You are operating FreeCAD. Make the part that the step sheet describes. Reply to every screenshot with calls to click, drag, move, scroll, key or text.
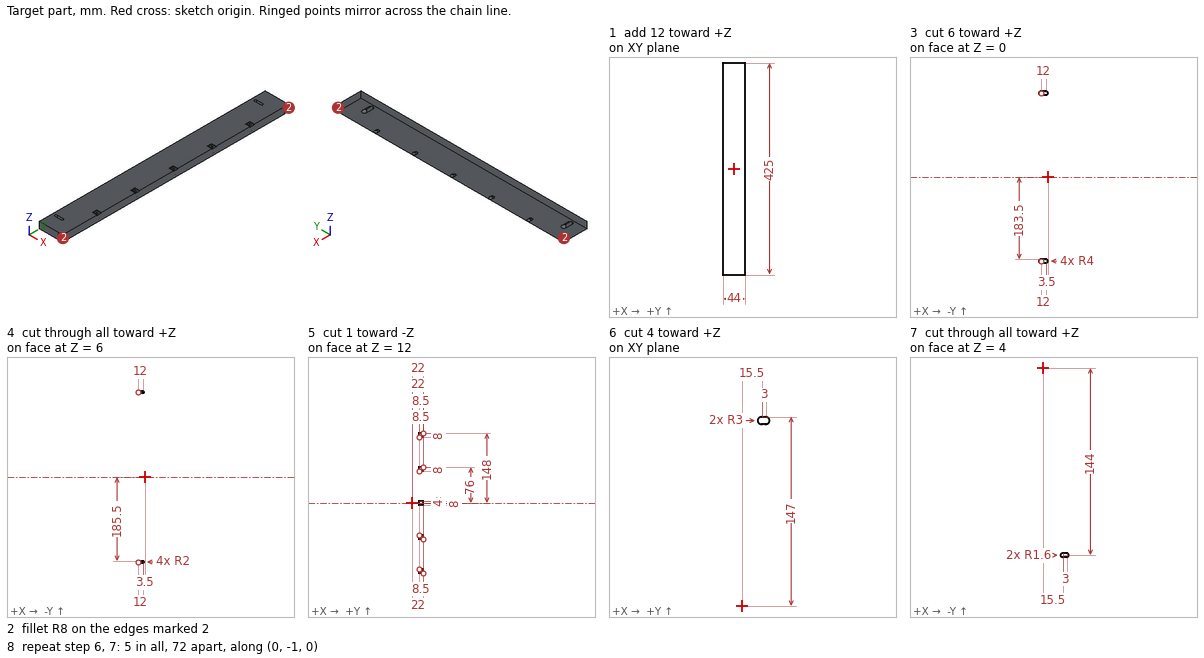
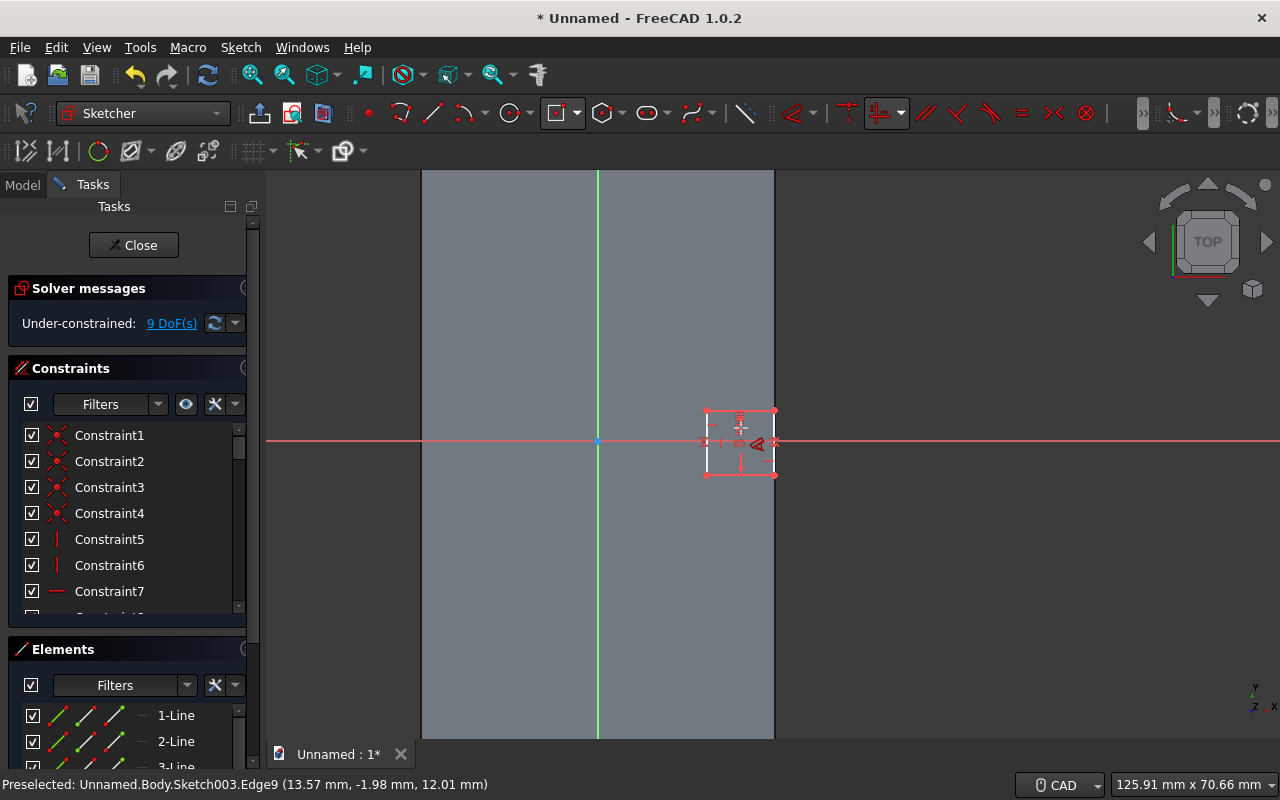
scroll(707, 411, up, 2)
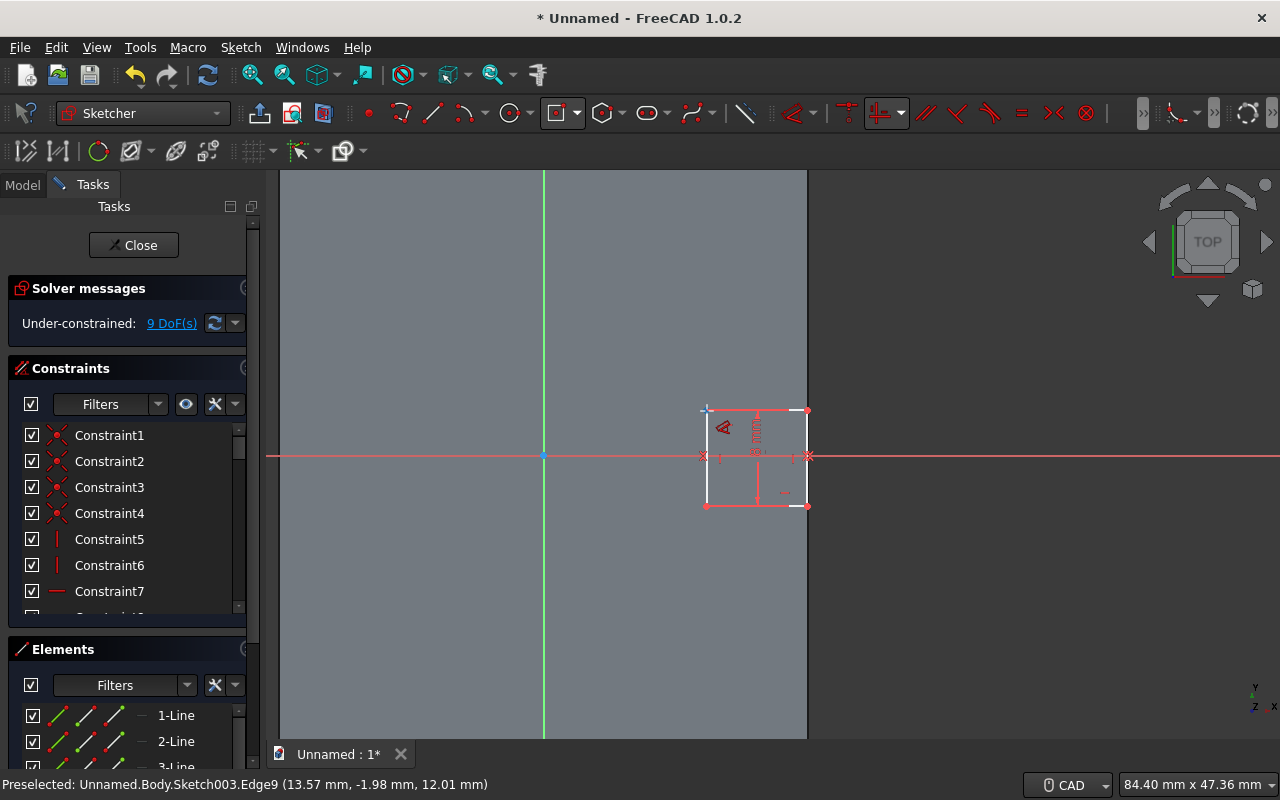
click(707, 410)
click(510, 433)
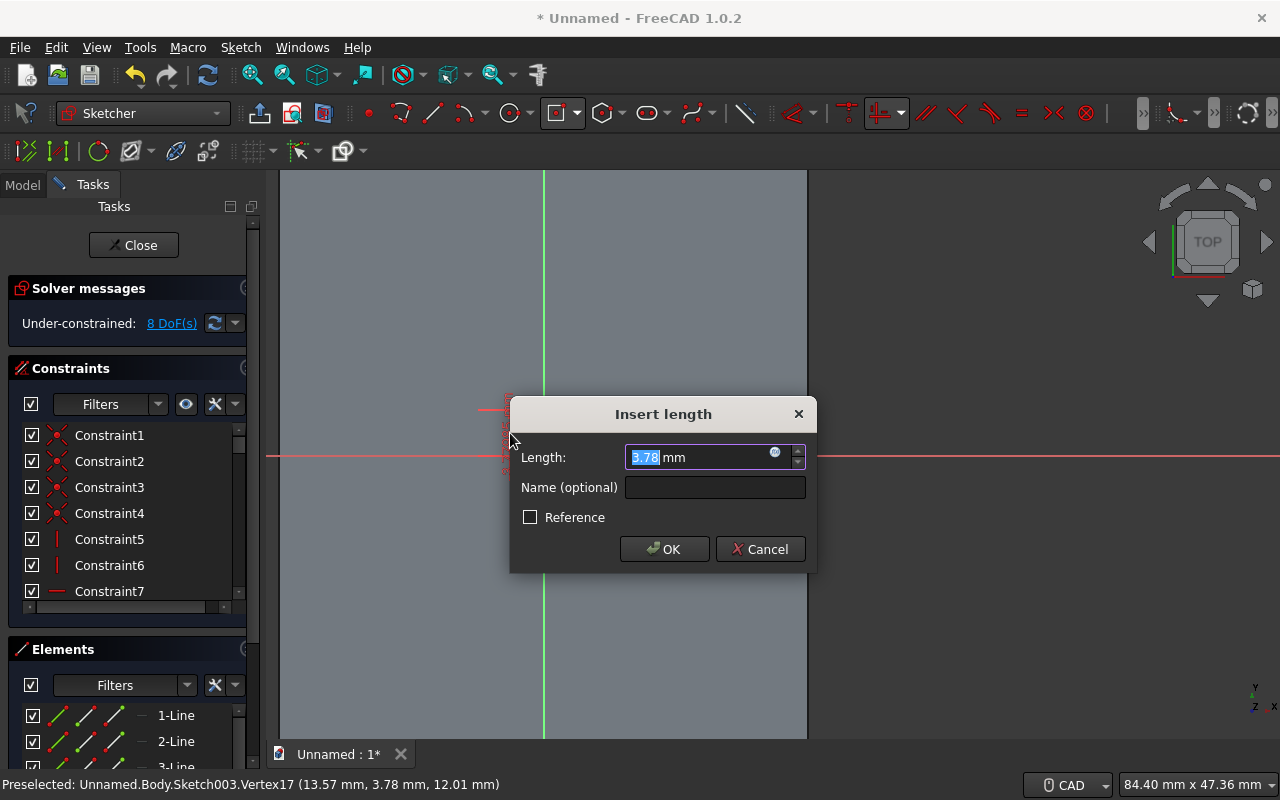
text(4)
key(Return)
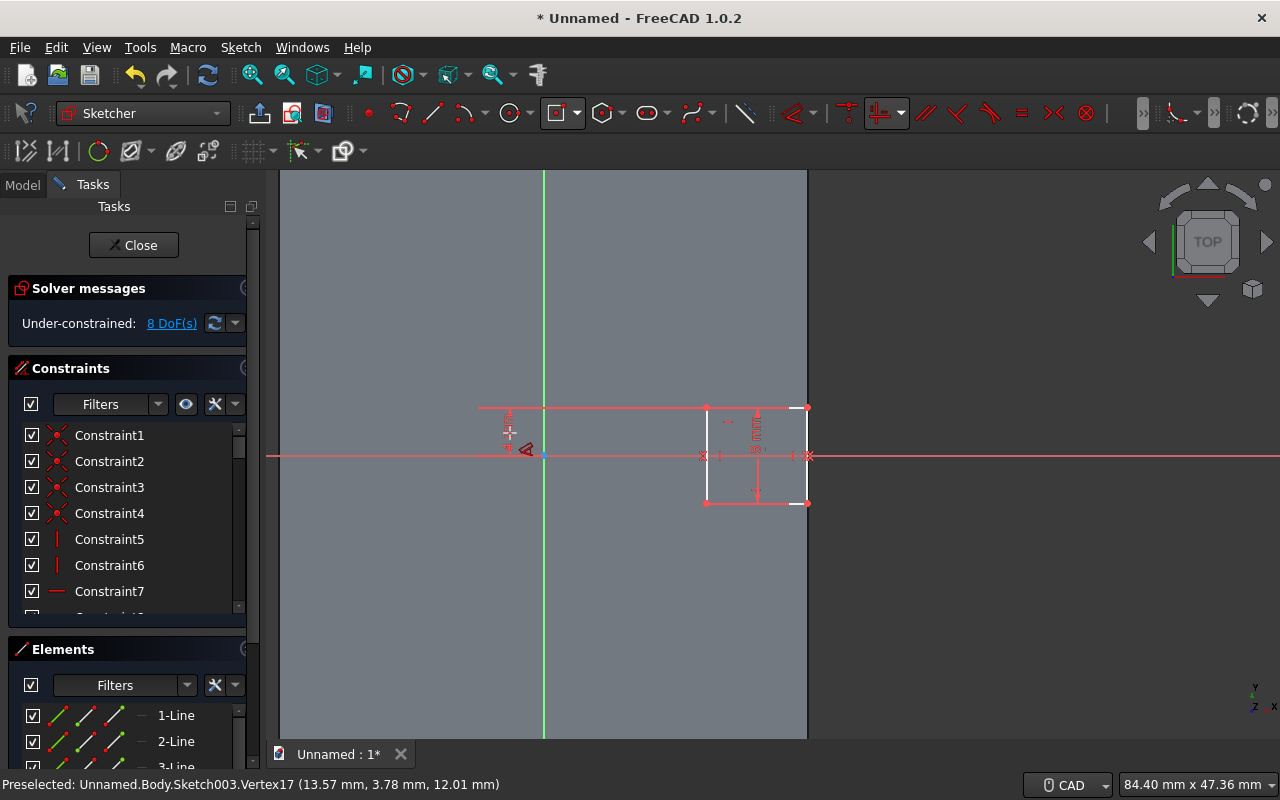
scroll(708, 454, down, 11)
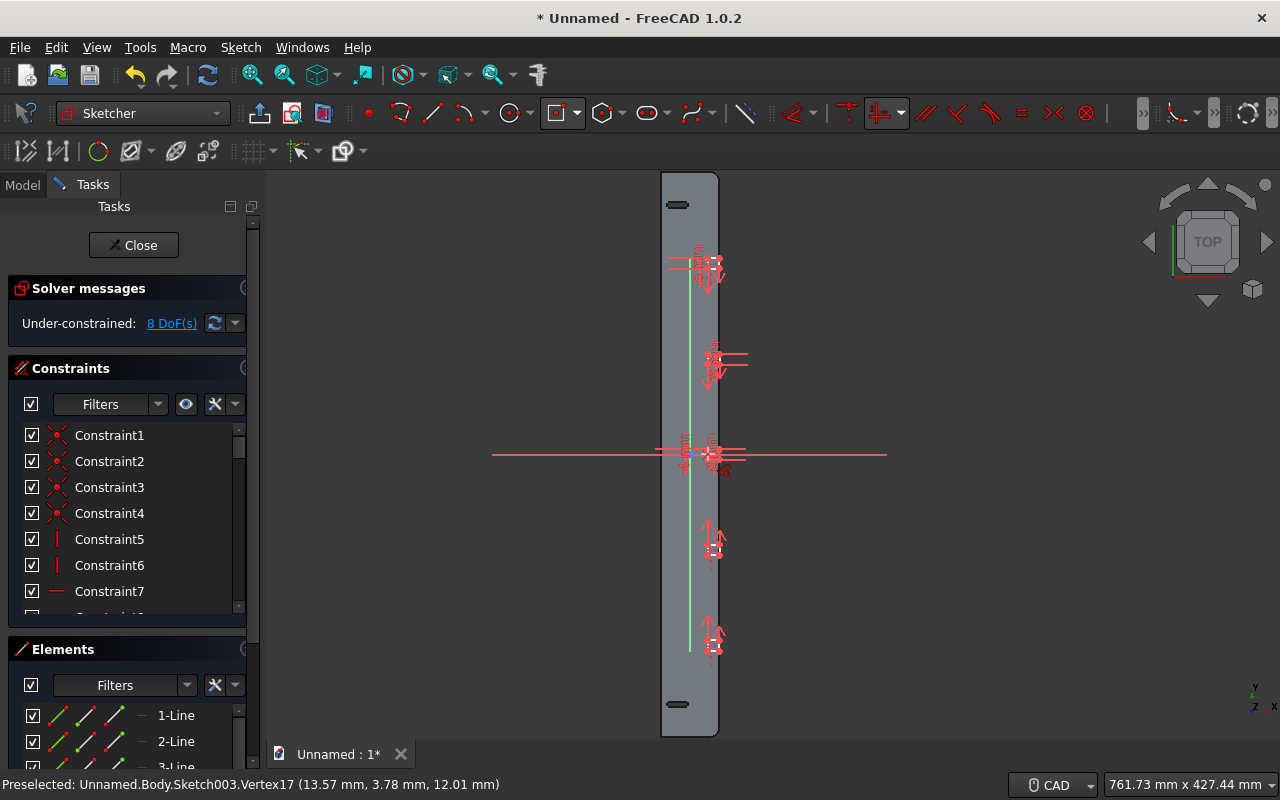
scroll(711, 269, up, 7)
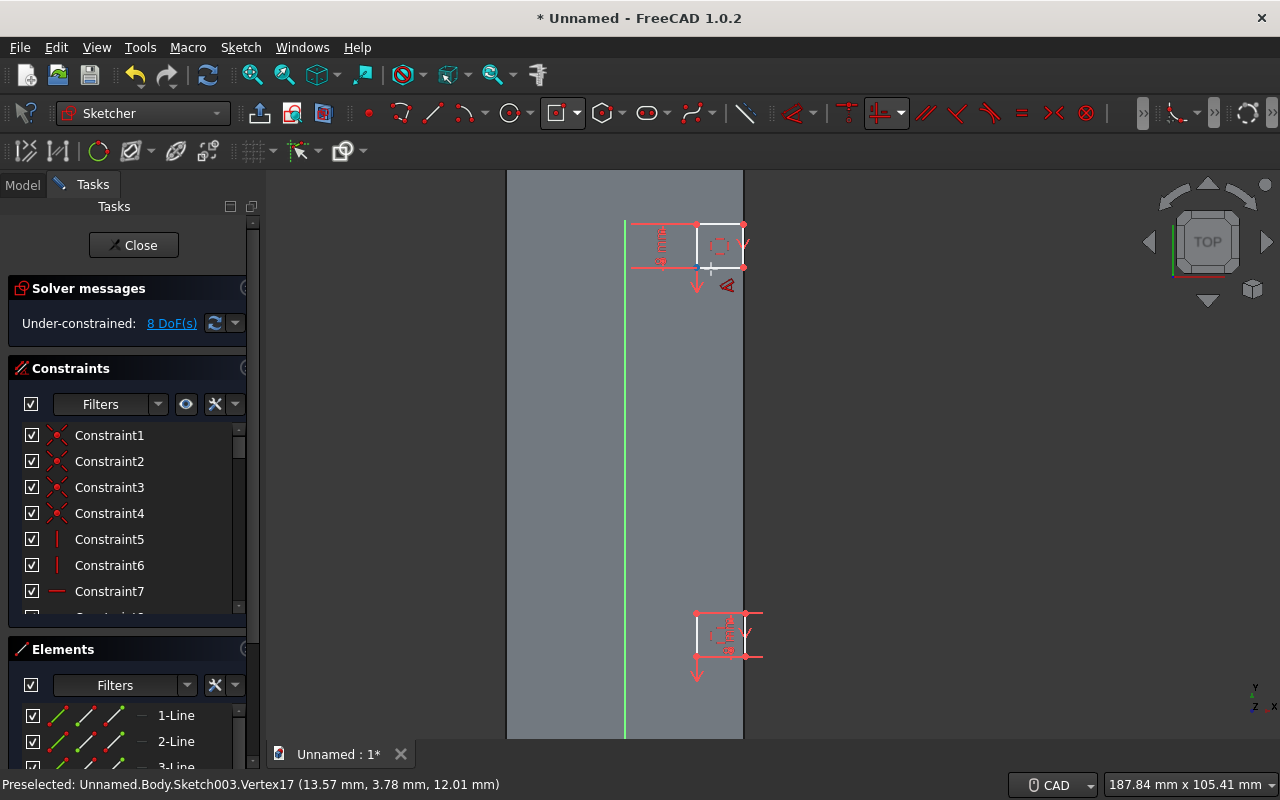
click(711, 268)
click(720, 302)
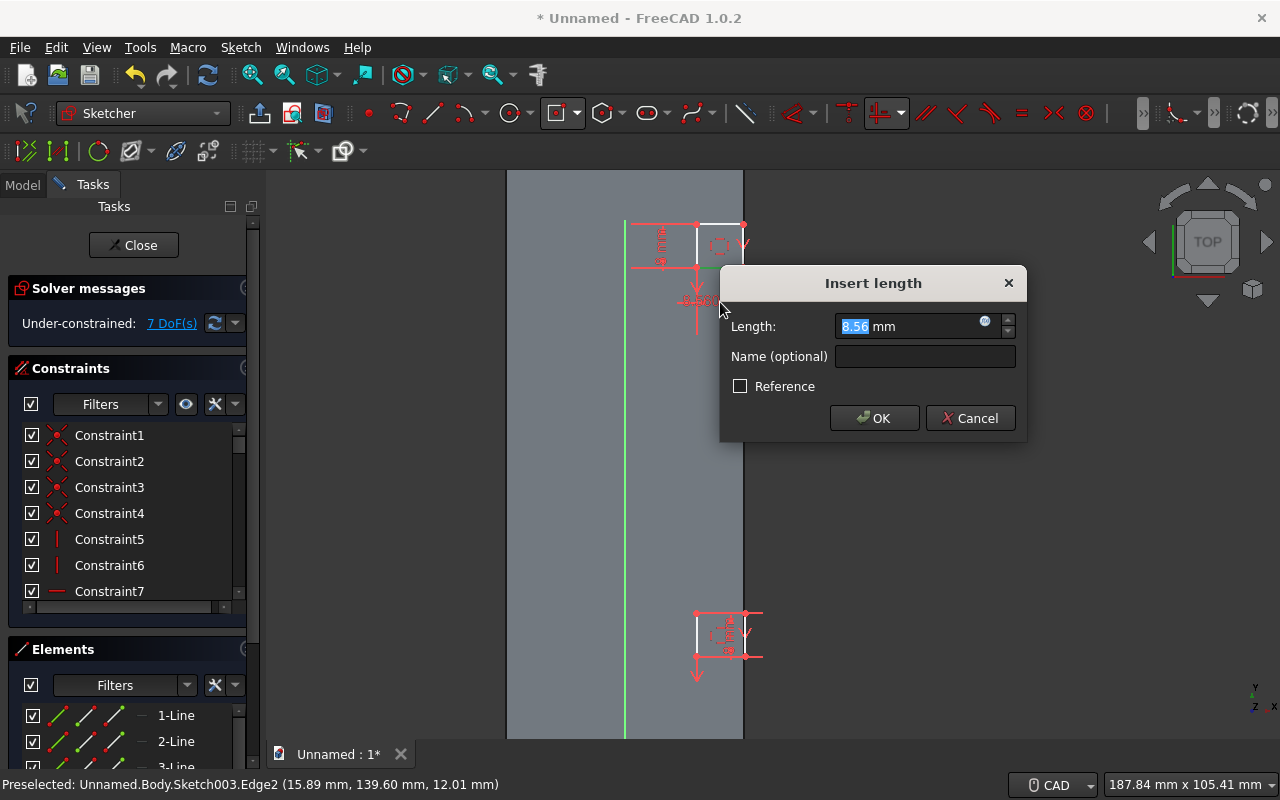
text(8.5)
key(Return)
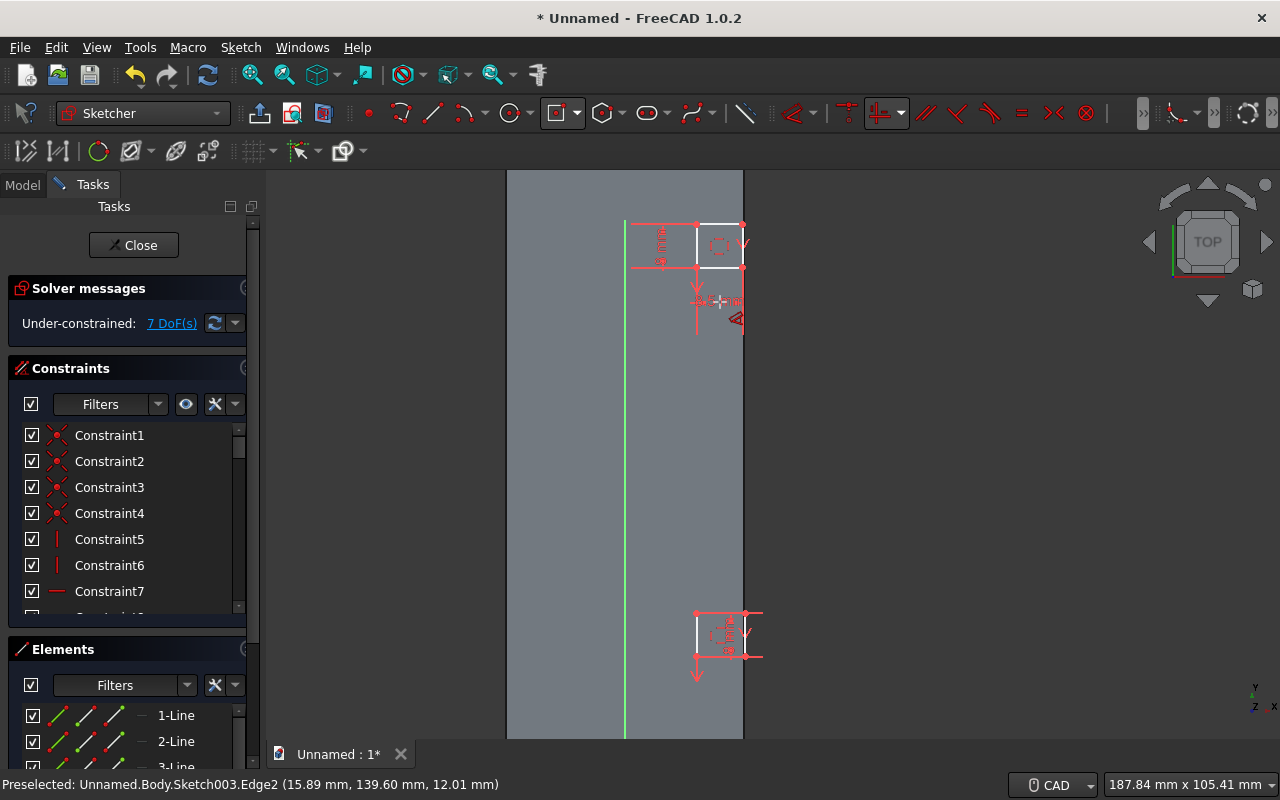
click(711, 657)
click(721, 691)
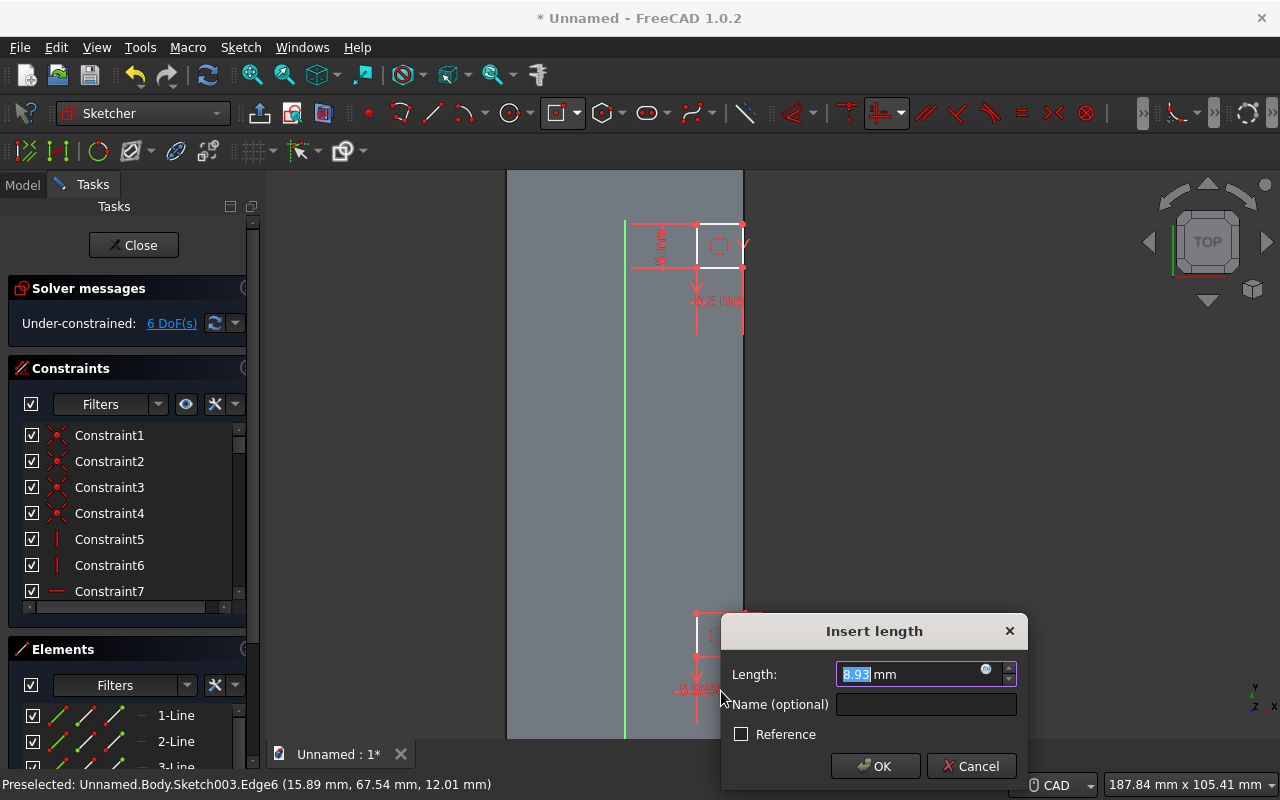
text(8.5)
key(Return)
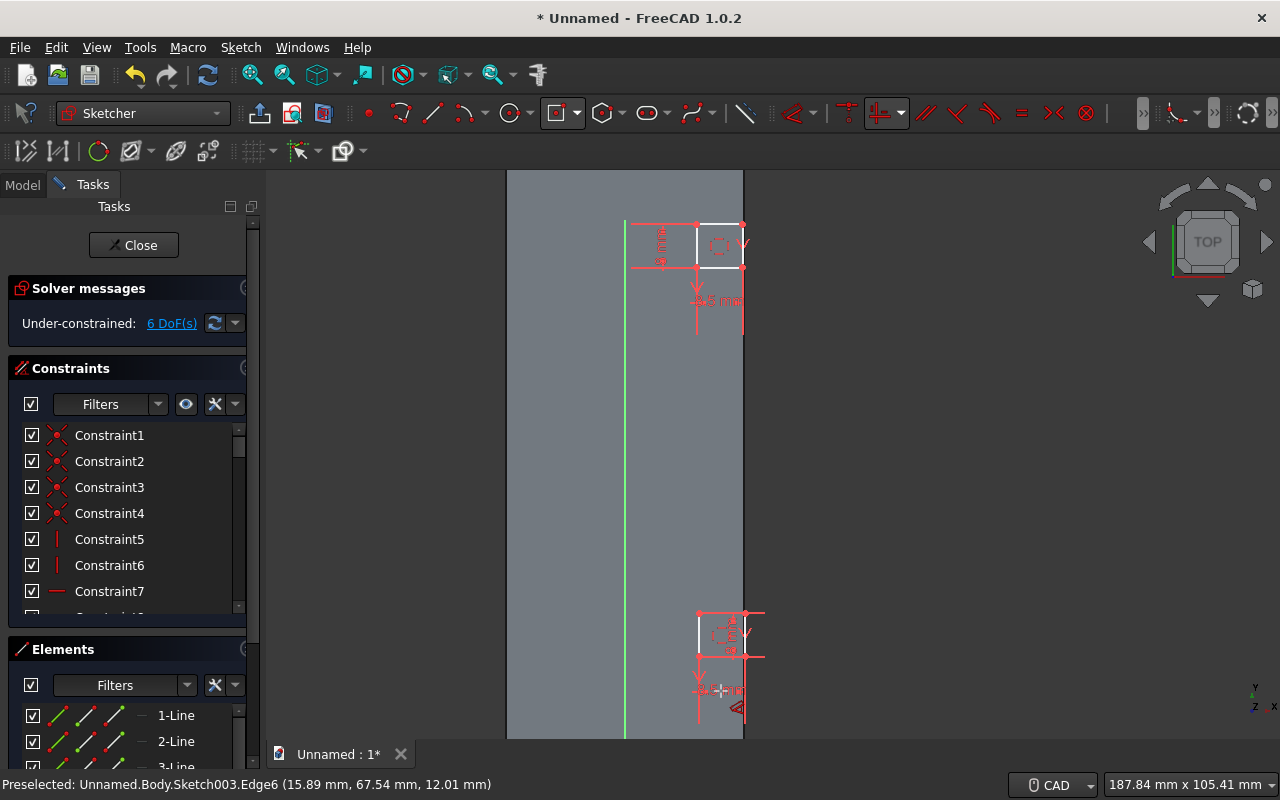
scroll(711, 269, down, 7)